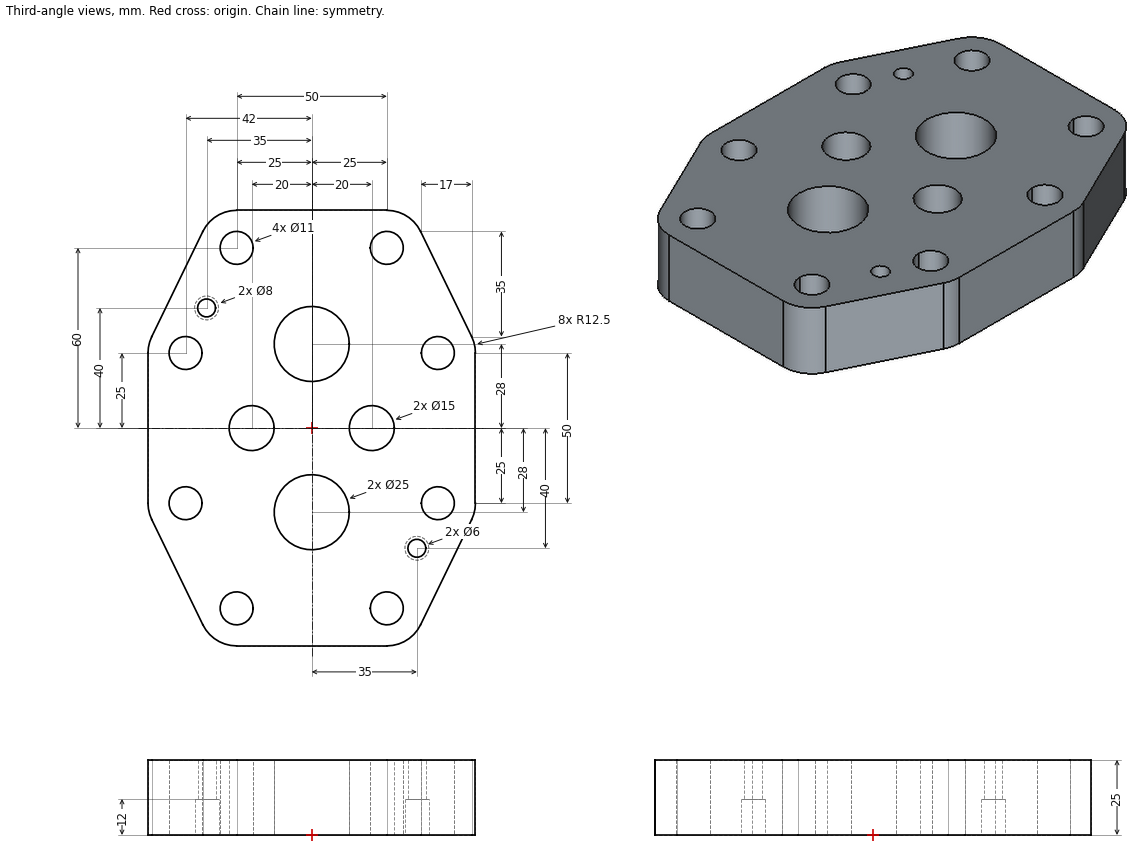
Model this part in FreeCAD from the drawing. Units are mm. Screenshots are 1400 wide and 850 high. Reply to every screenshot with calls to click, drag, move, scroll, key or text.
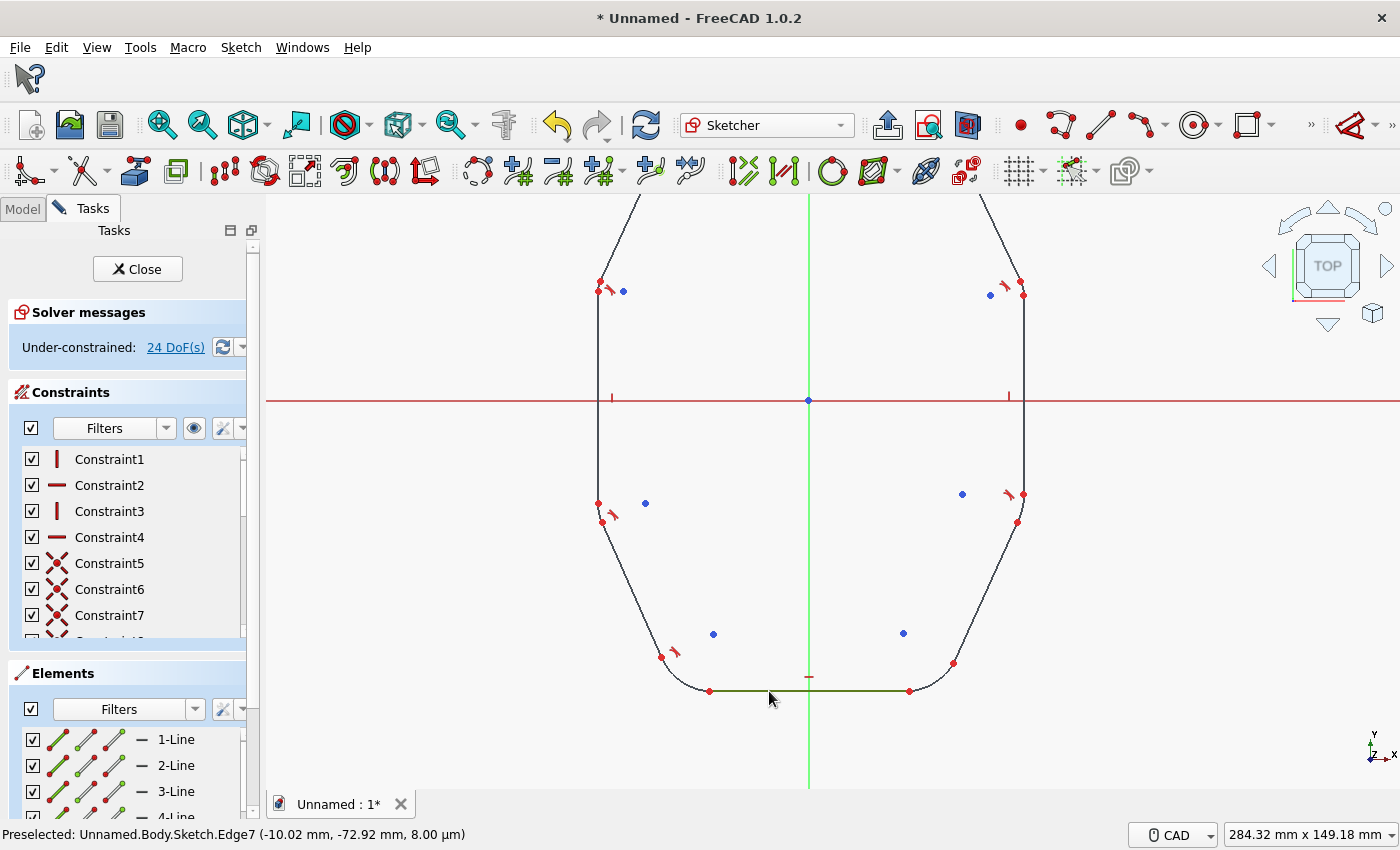
click(672, 673)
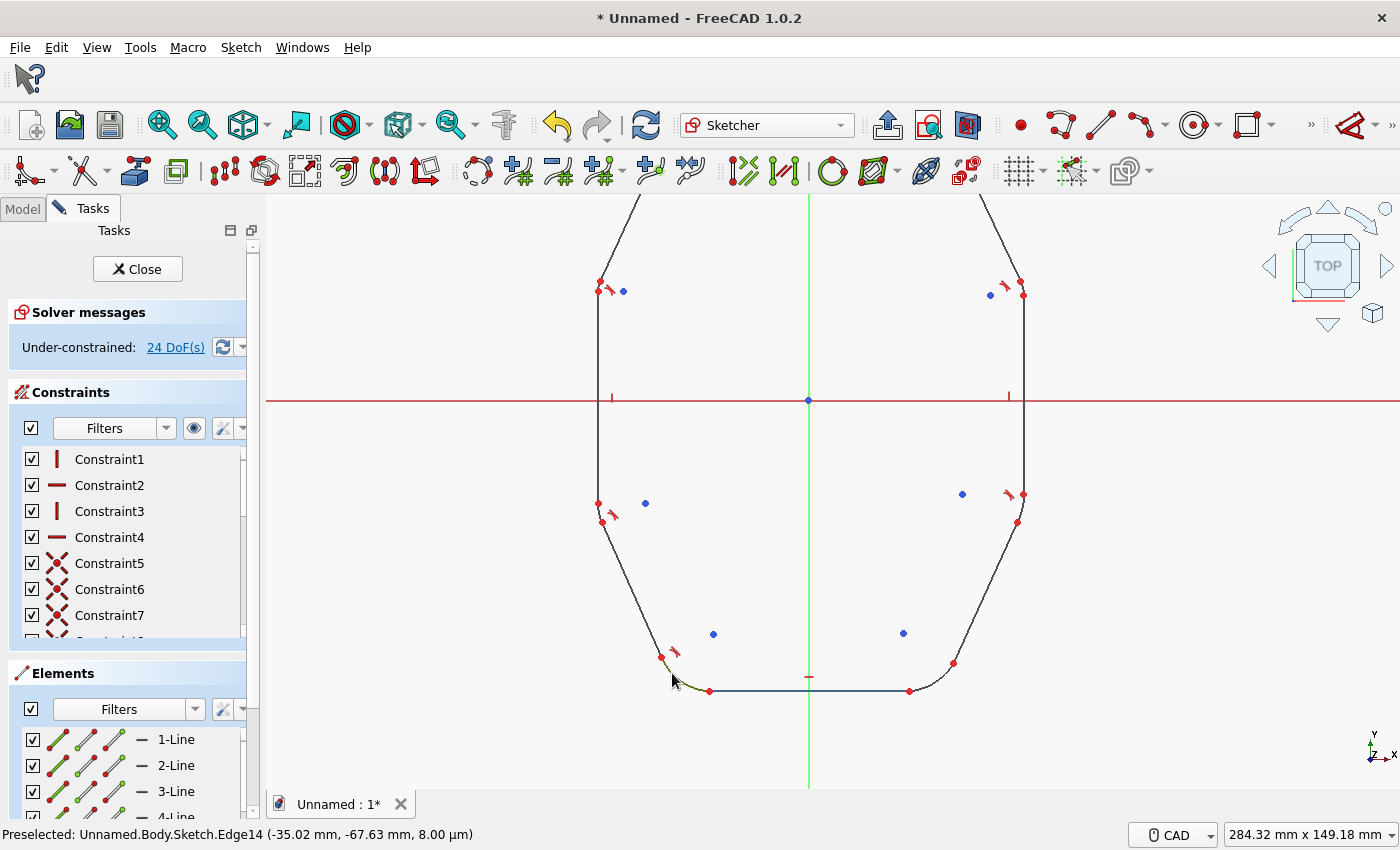
key(t)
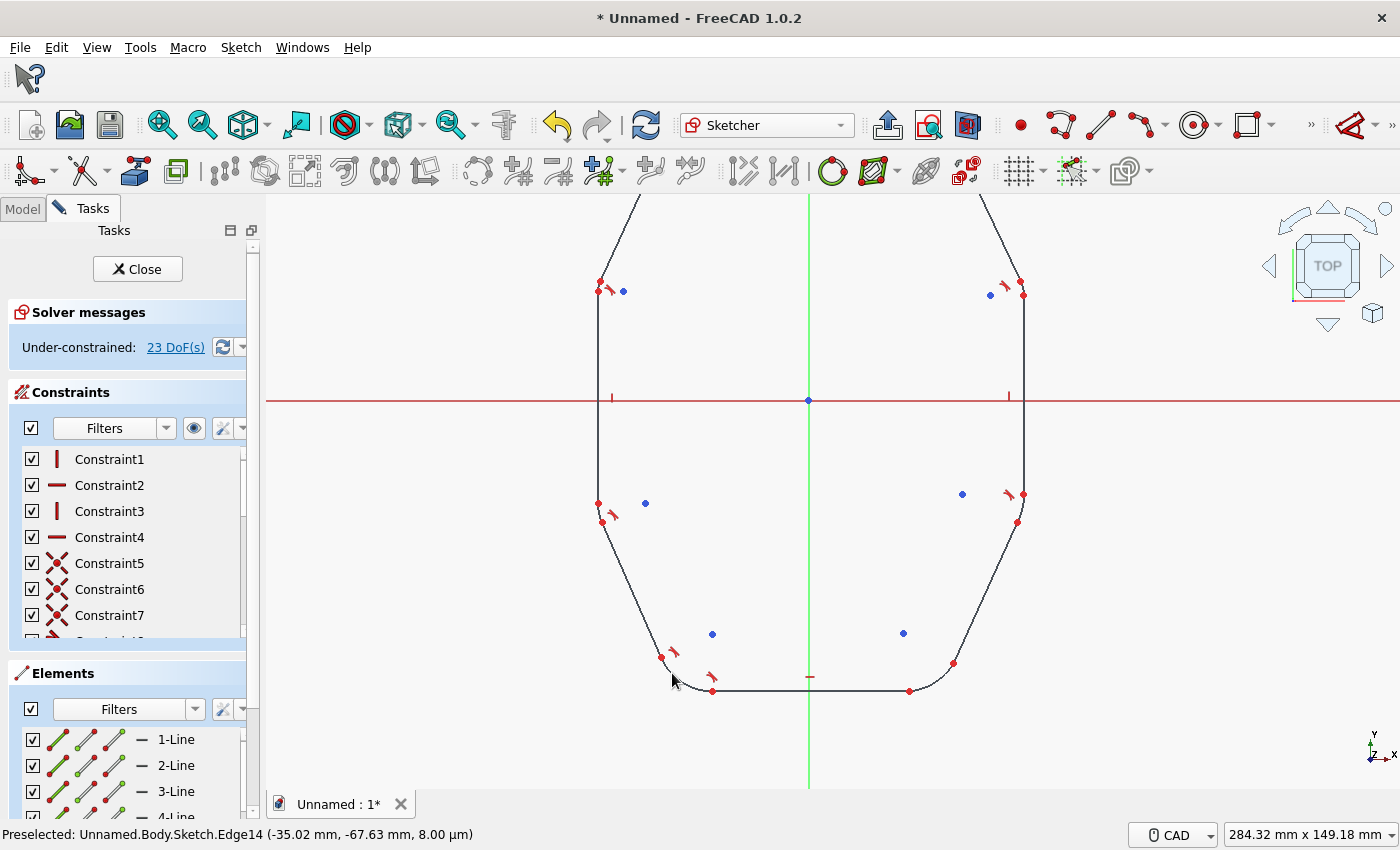
click(772, 691)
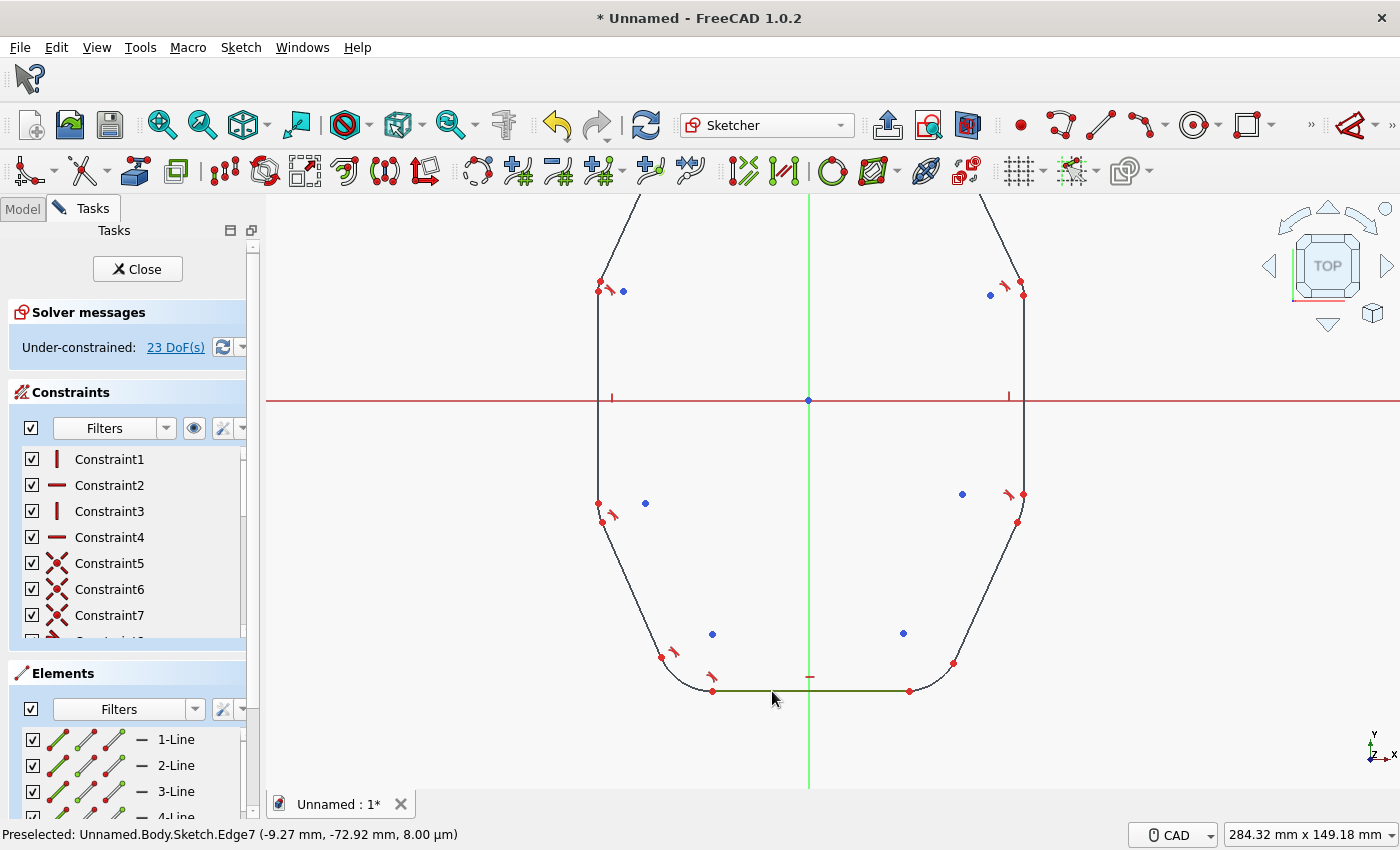
click(925, 688)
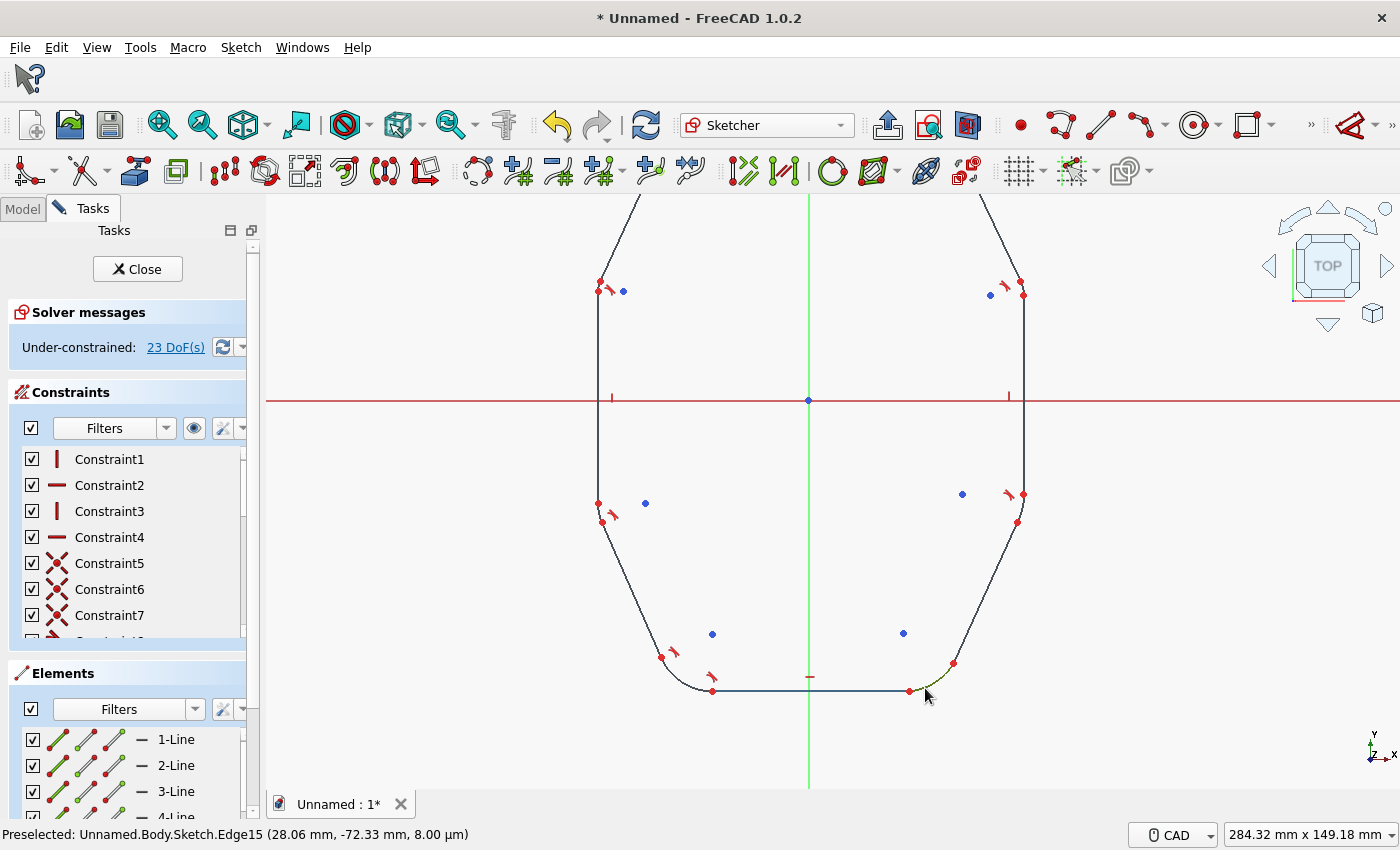
key(t)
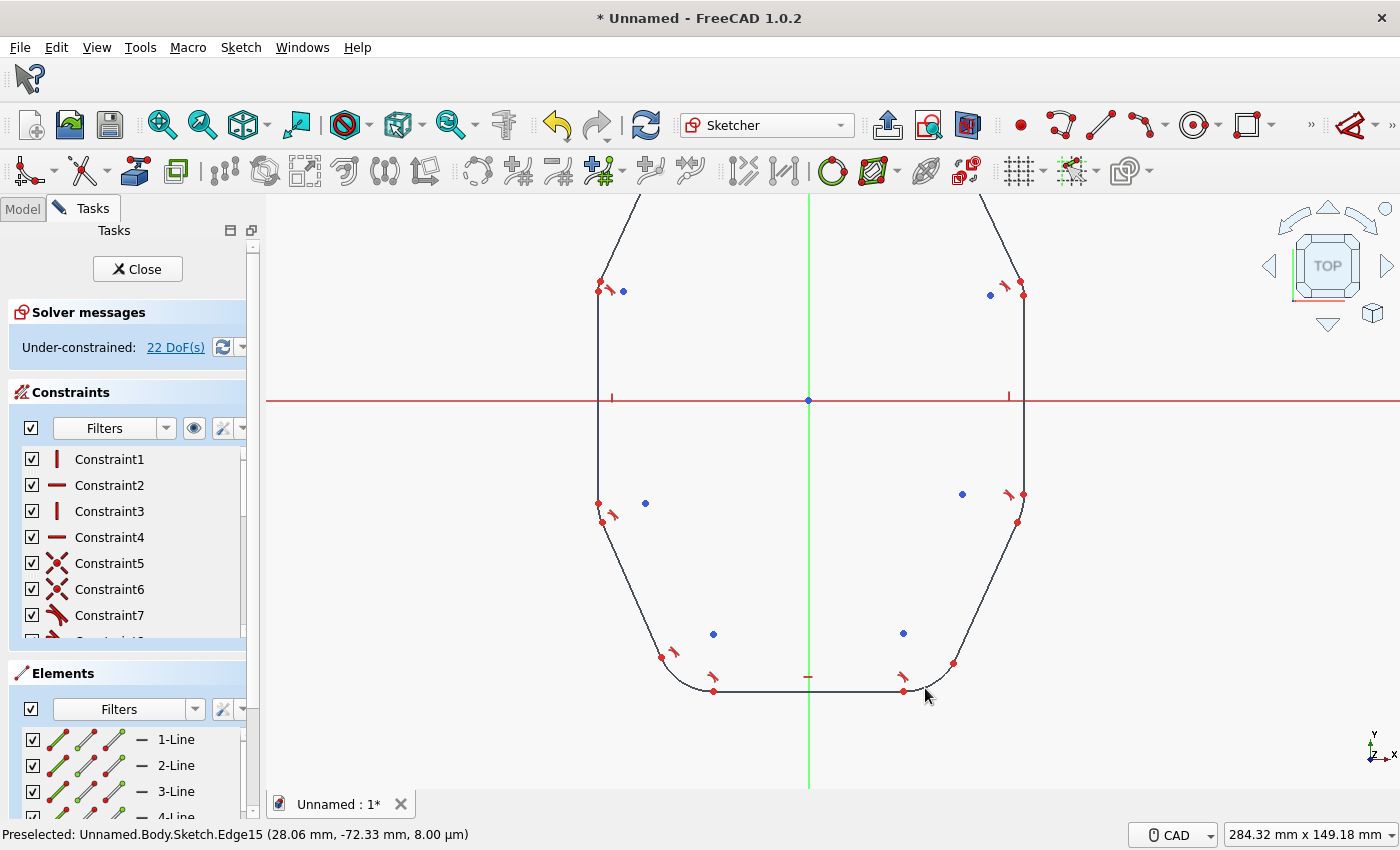
click(973, 621)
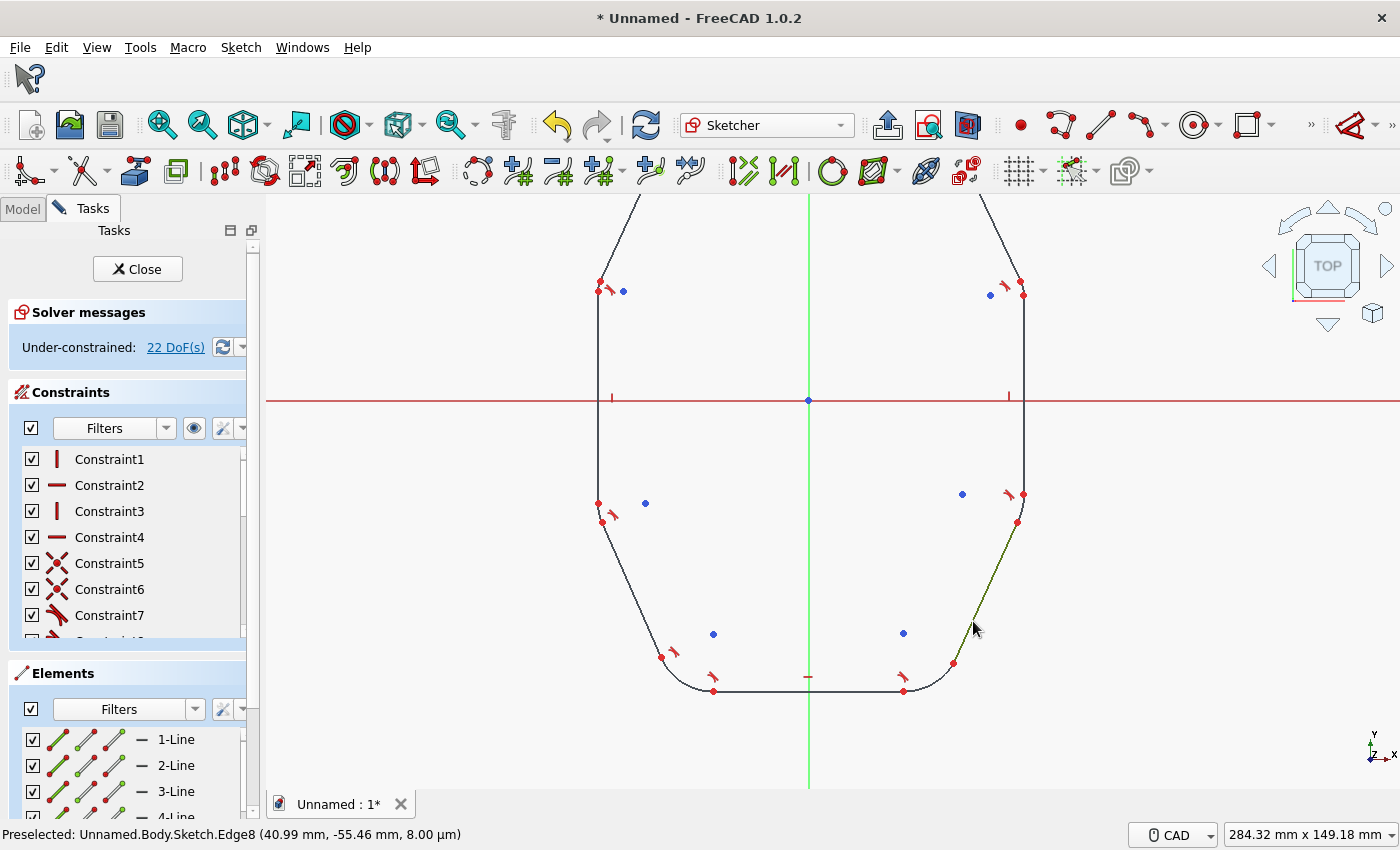
click(922, 689)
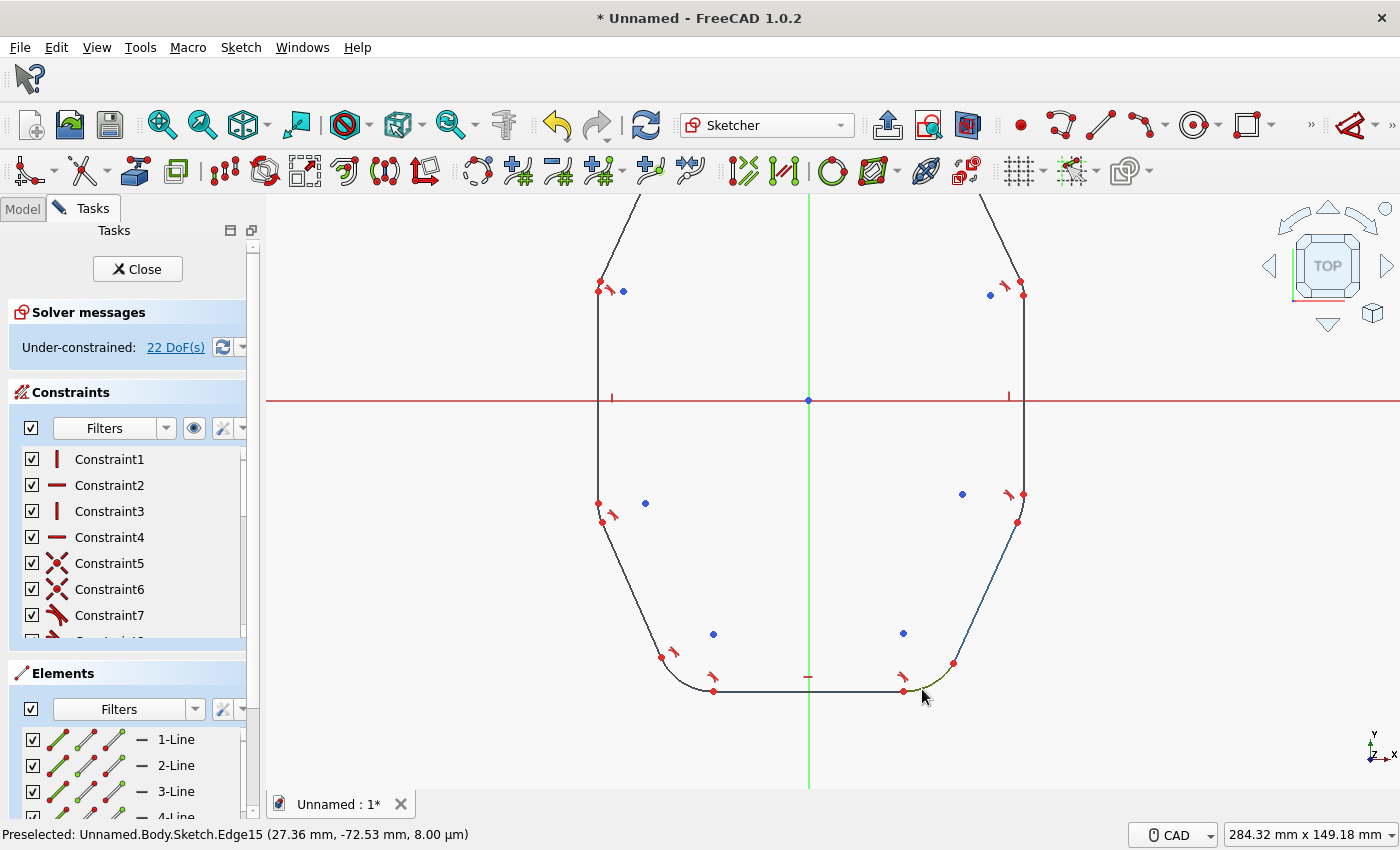
key(t)